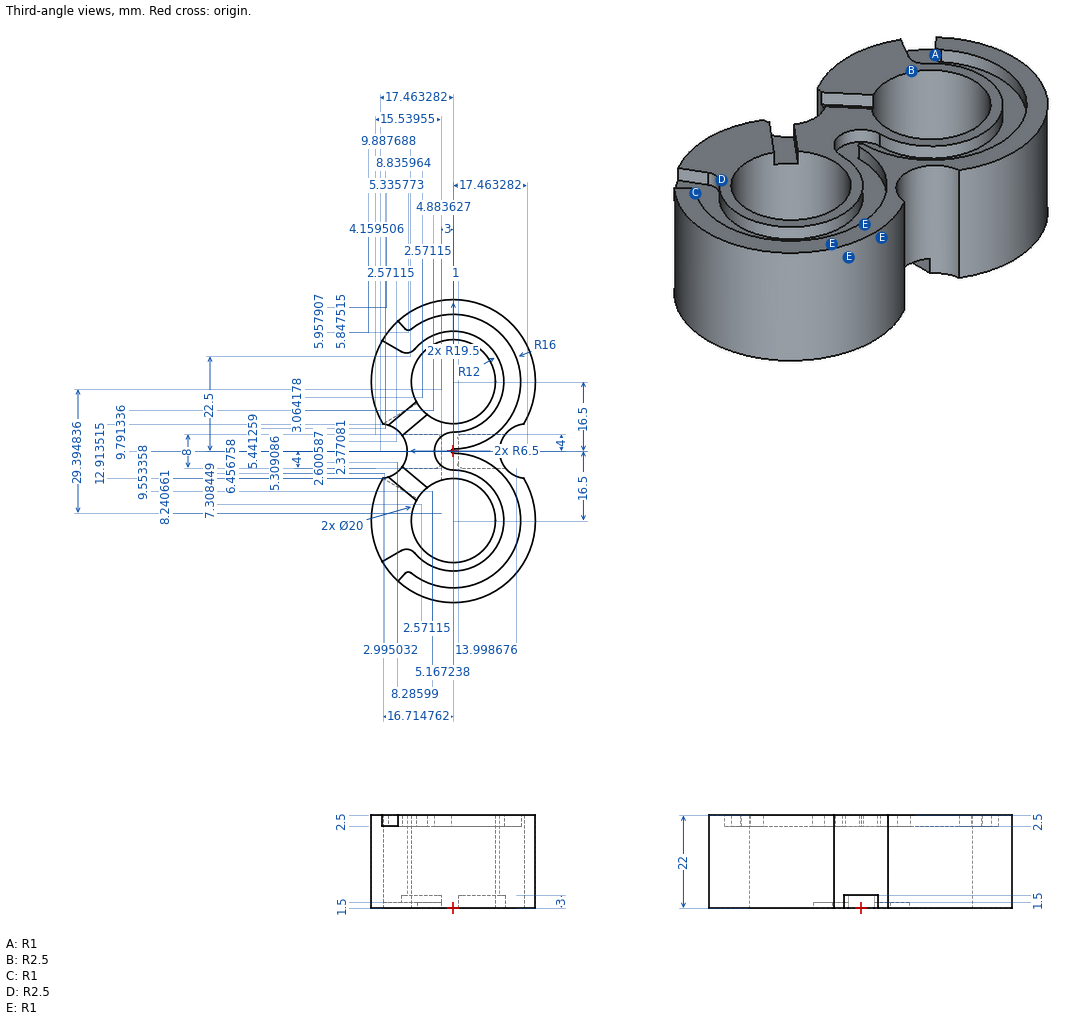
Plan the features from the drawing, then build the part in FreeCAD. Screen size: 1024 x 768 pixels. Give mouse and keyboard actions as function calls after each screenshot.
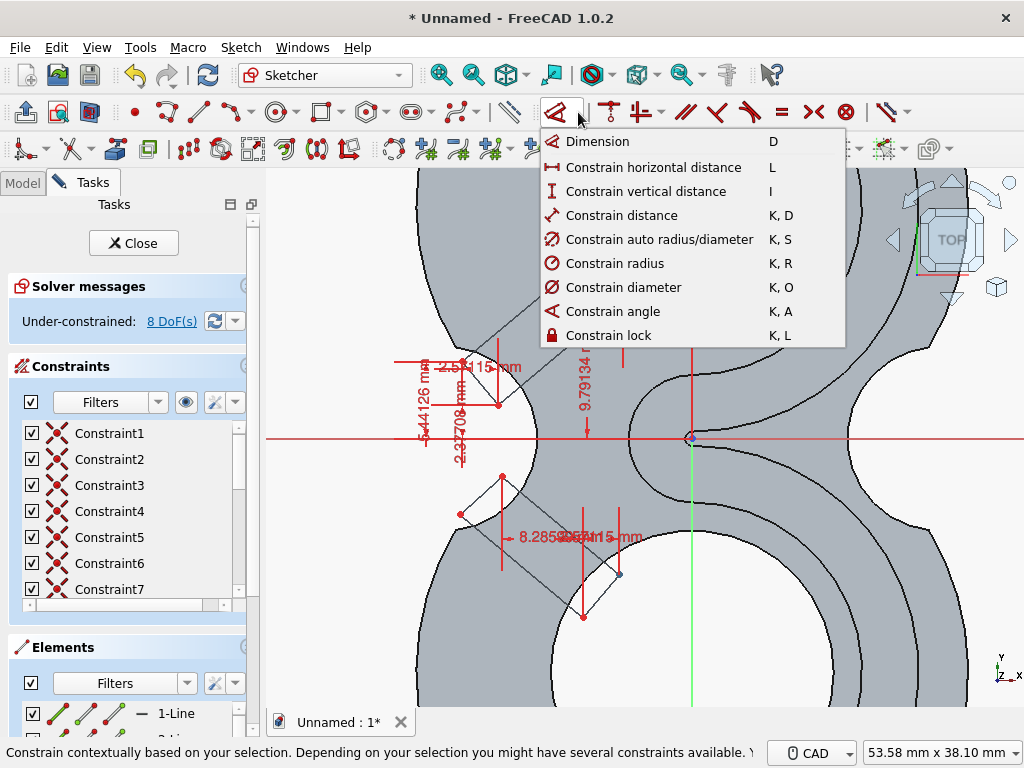
click(693, 167)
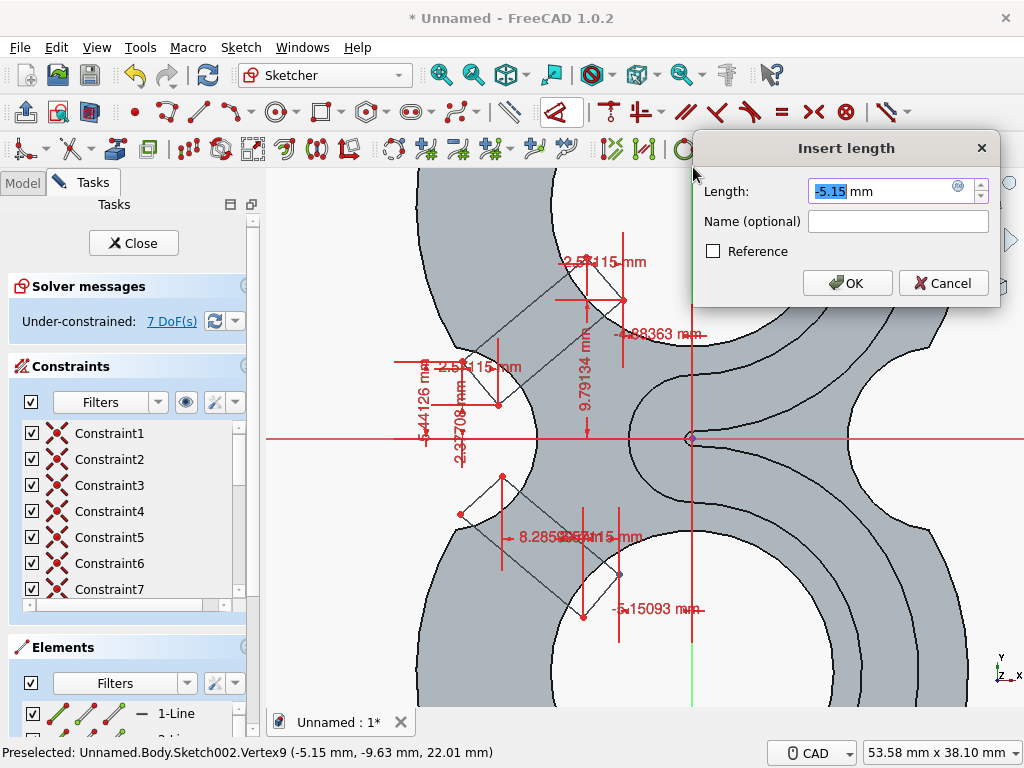
text(-5.167238)
key(Return)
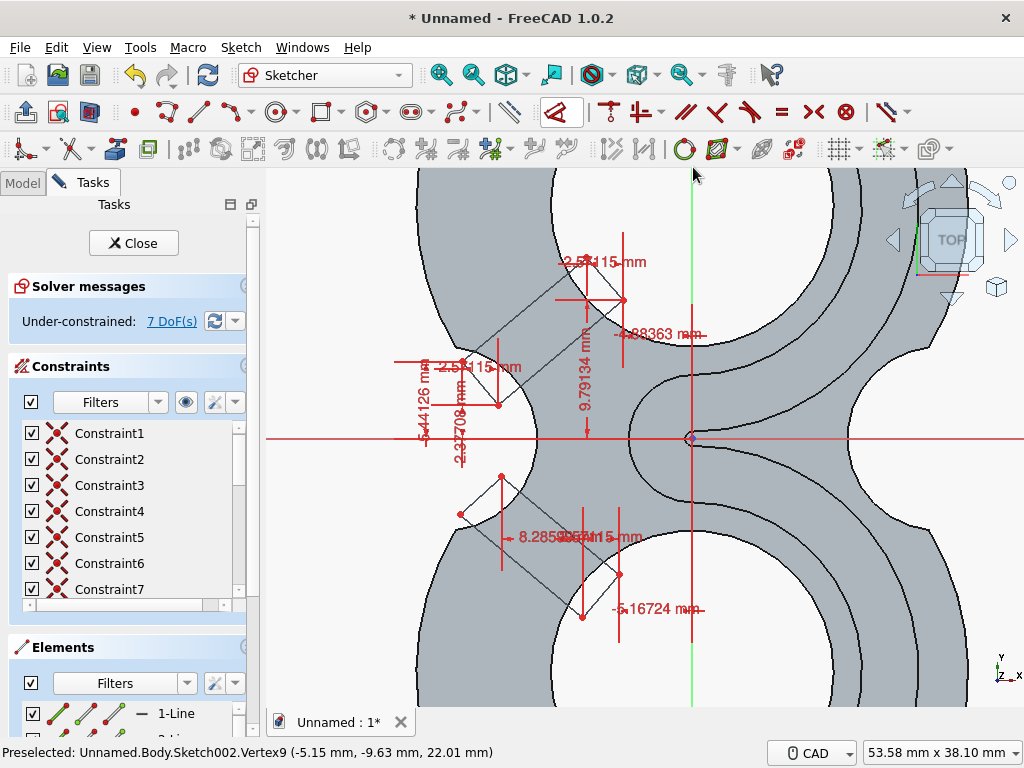
click(619, 575)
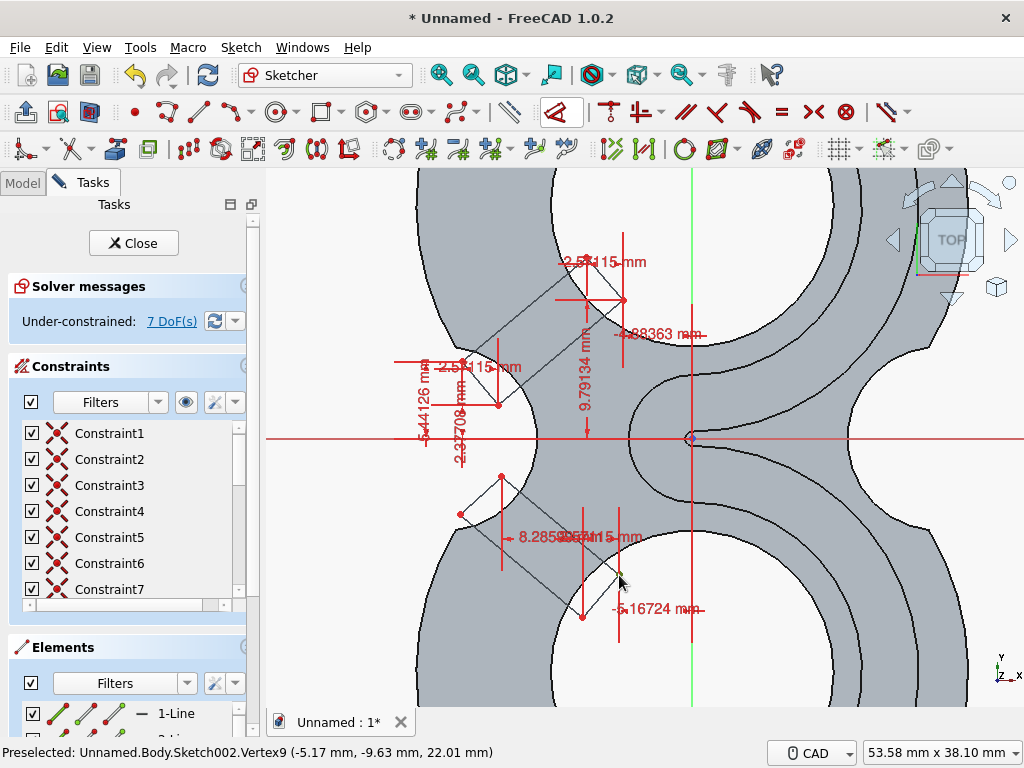
click(578, 112)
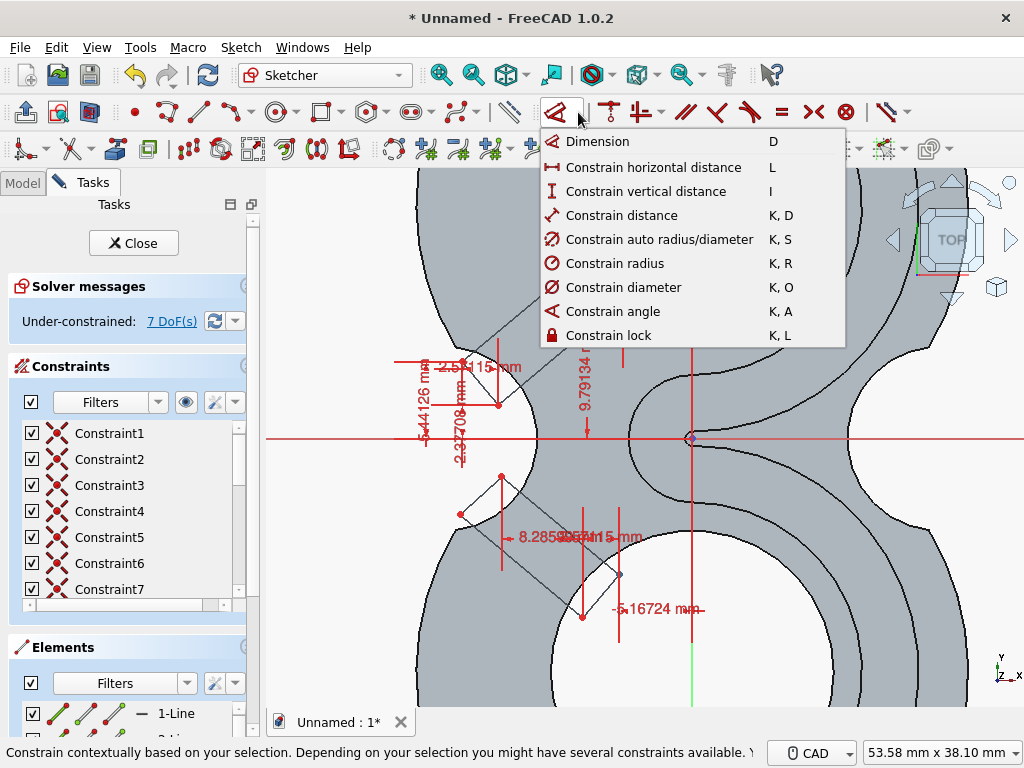
click(693, 191)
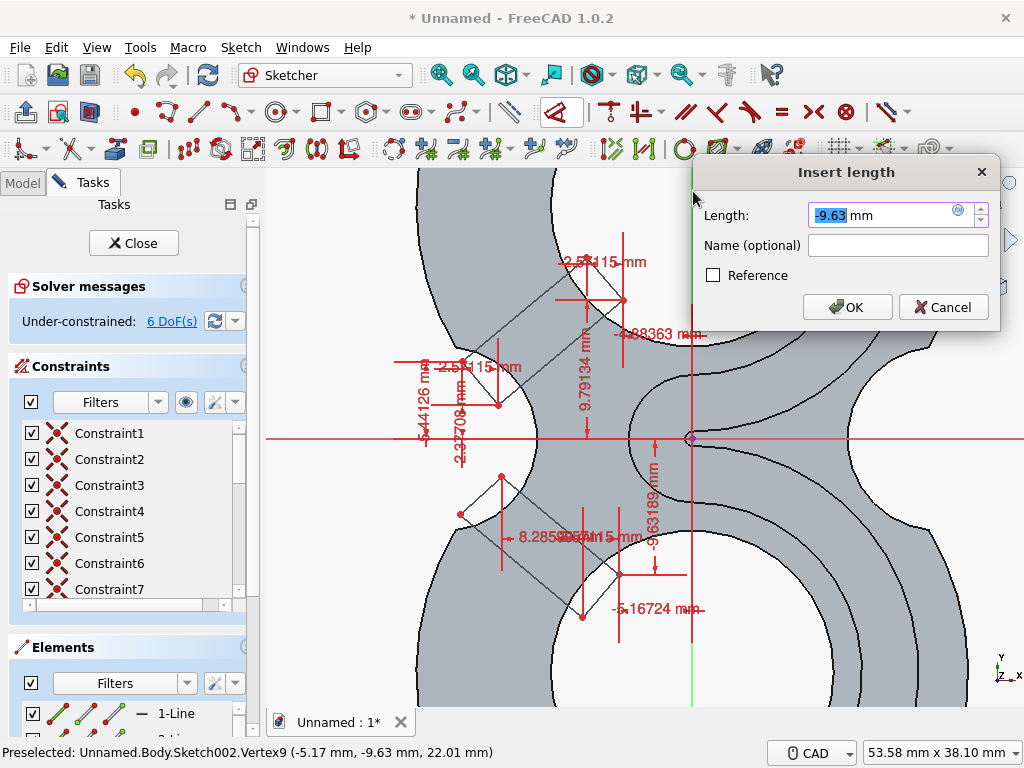
text(-9.553358)
key(Return)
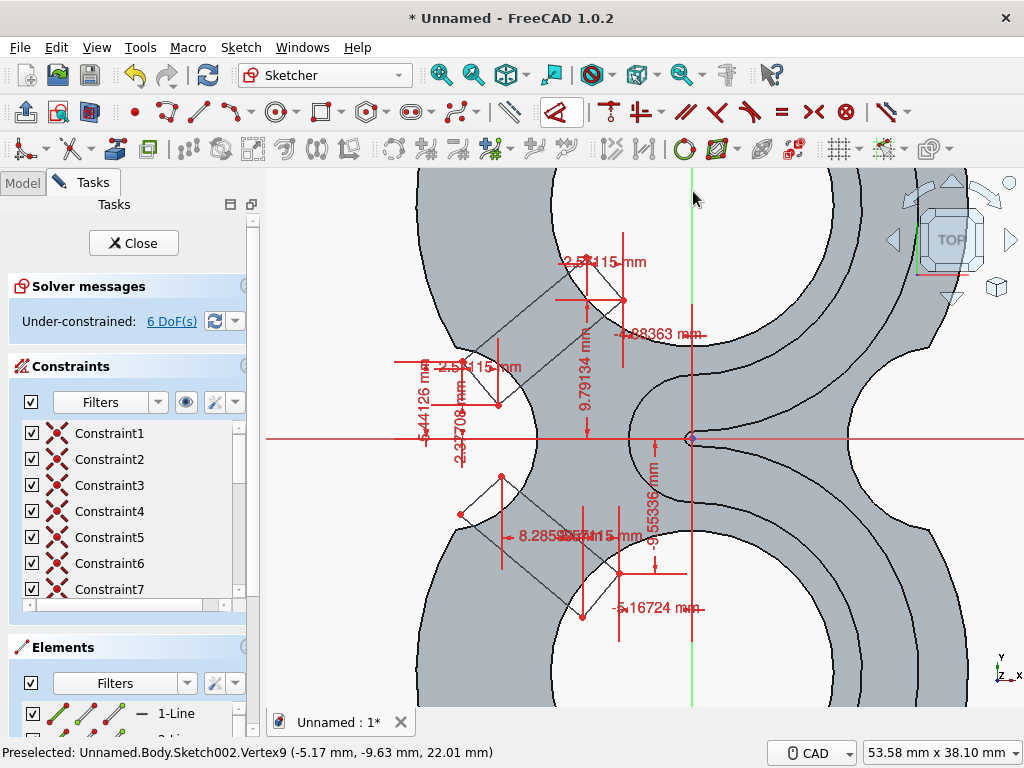
click(502, 477)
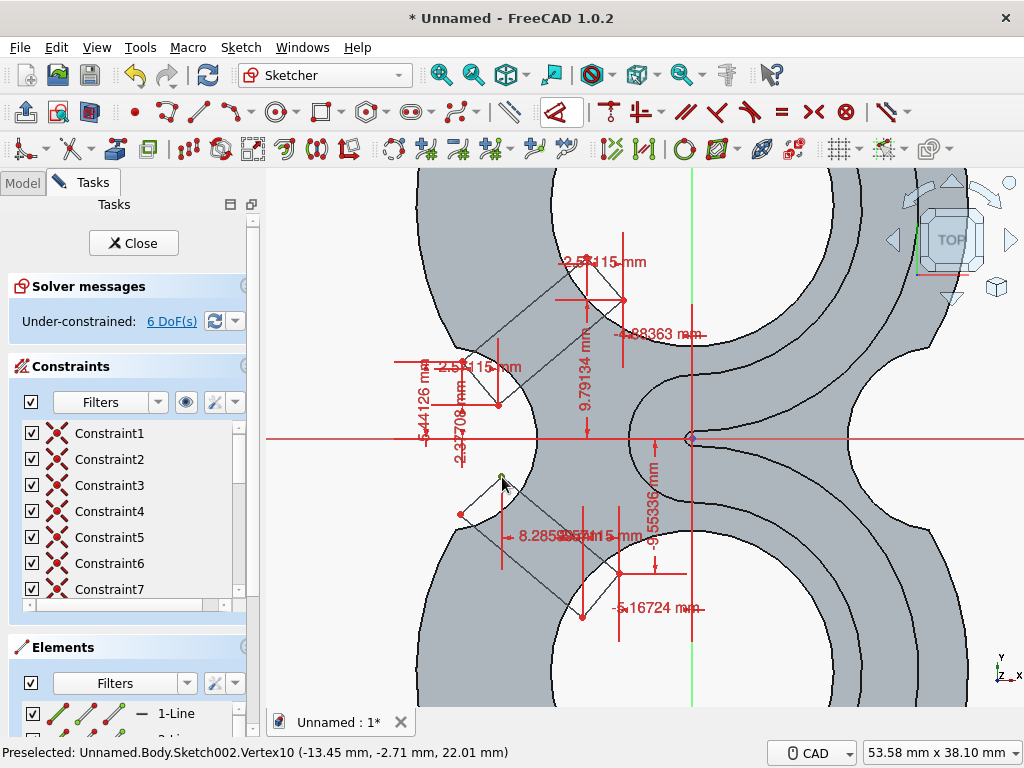
key(i)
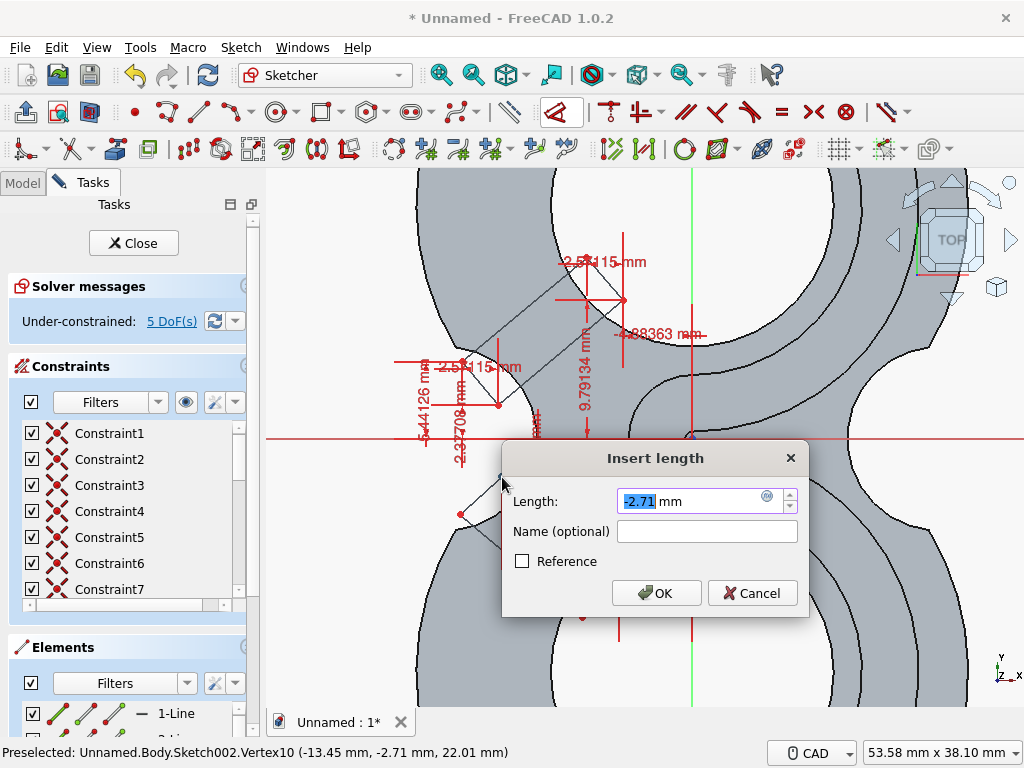
text(-2.600587)
key(Return)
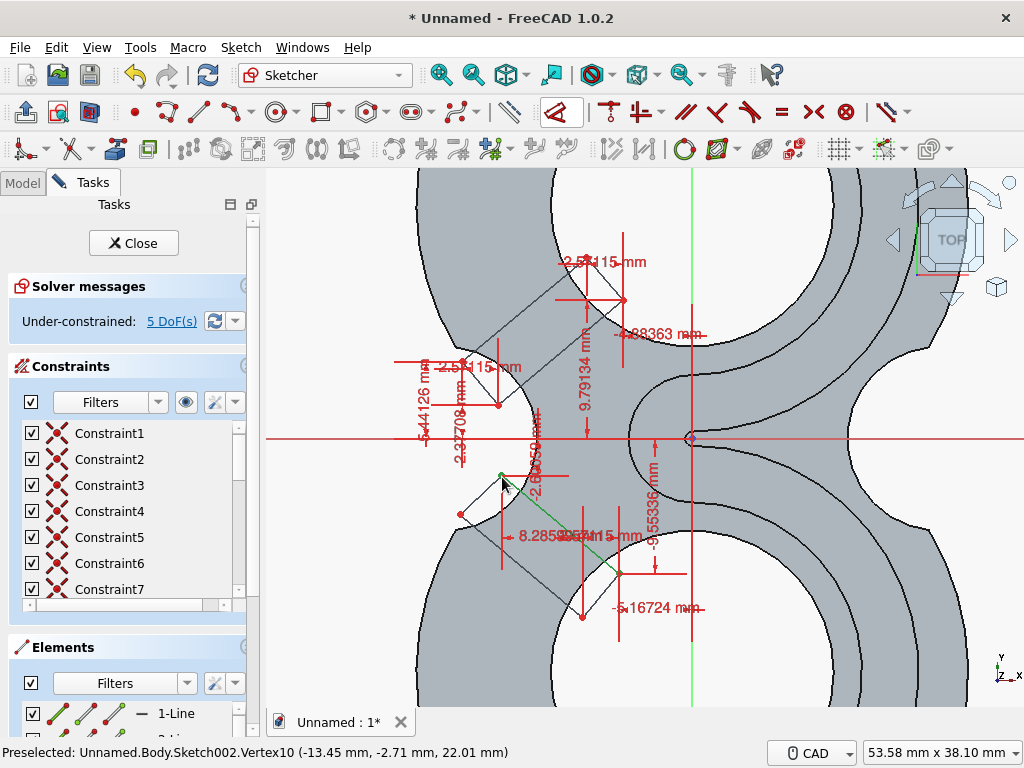
click(460, 515)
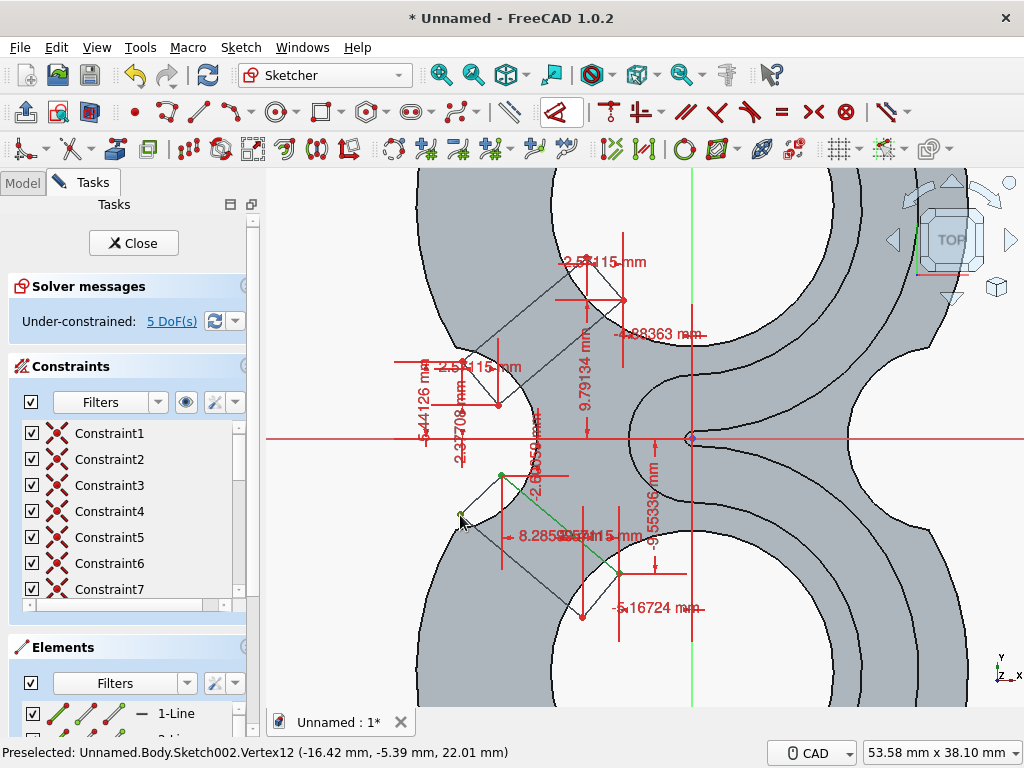
key(i)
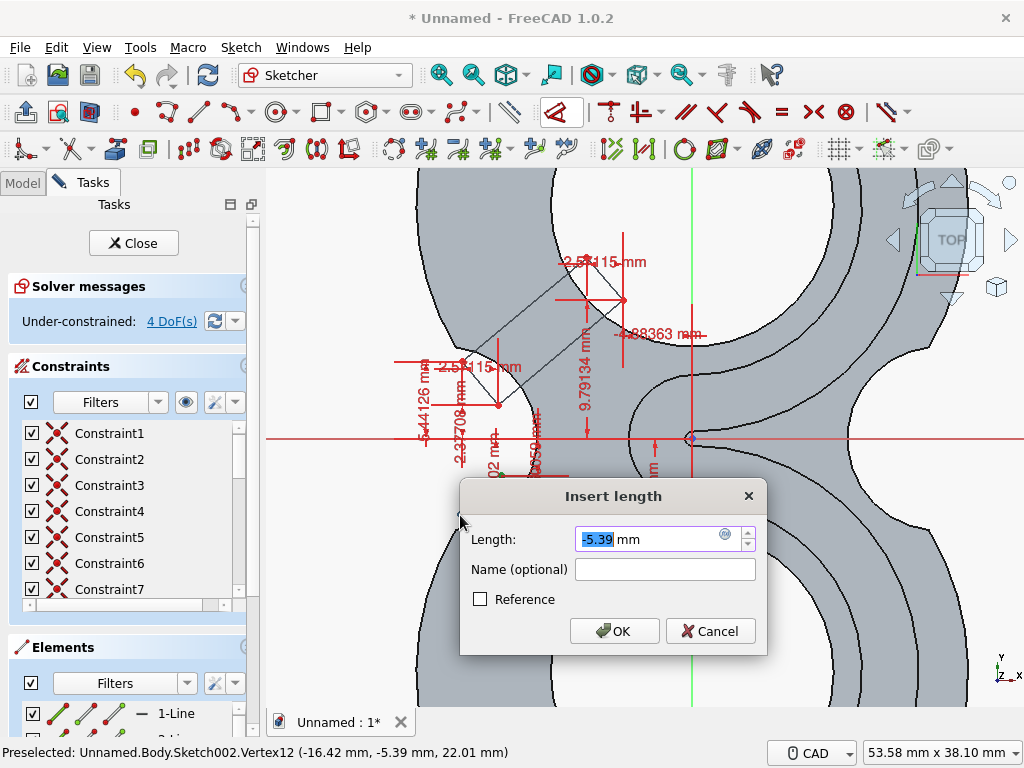
text(-5.309086)
key(Return)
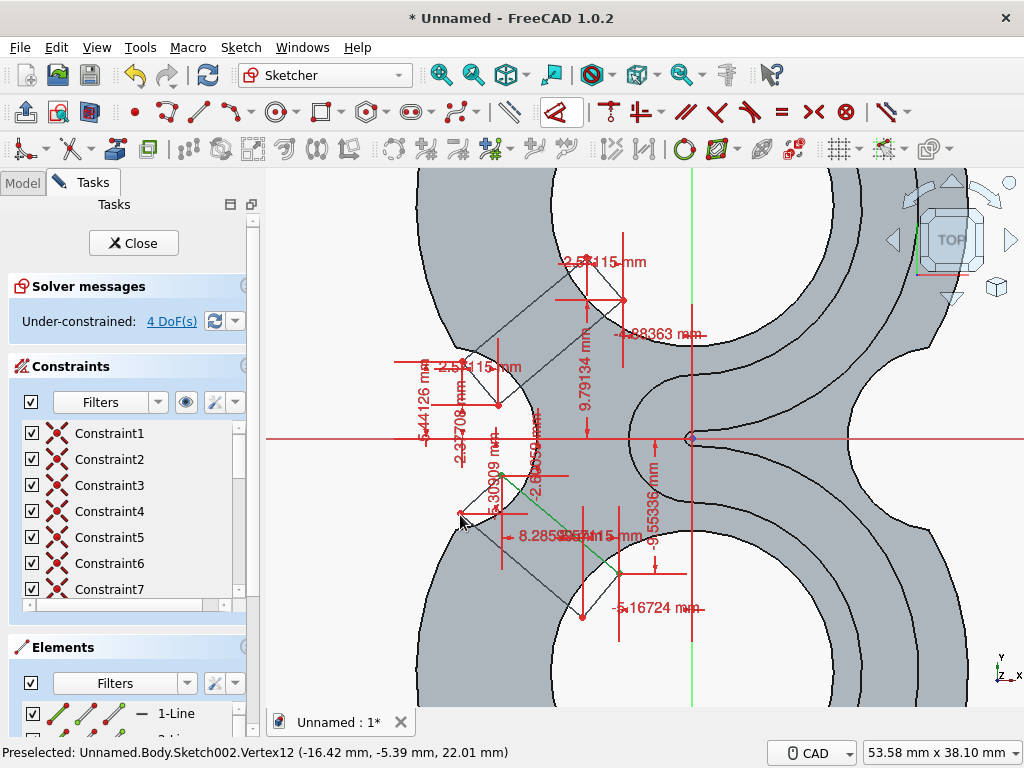
click(612, 288)